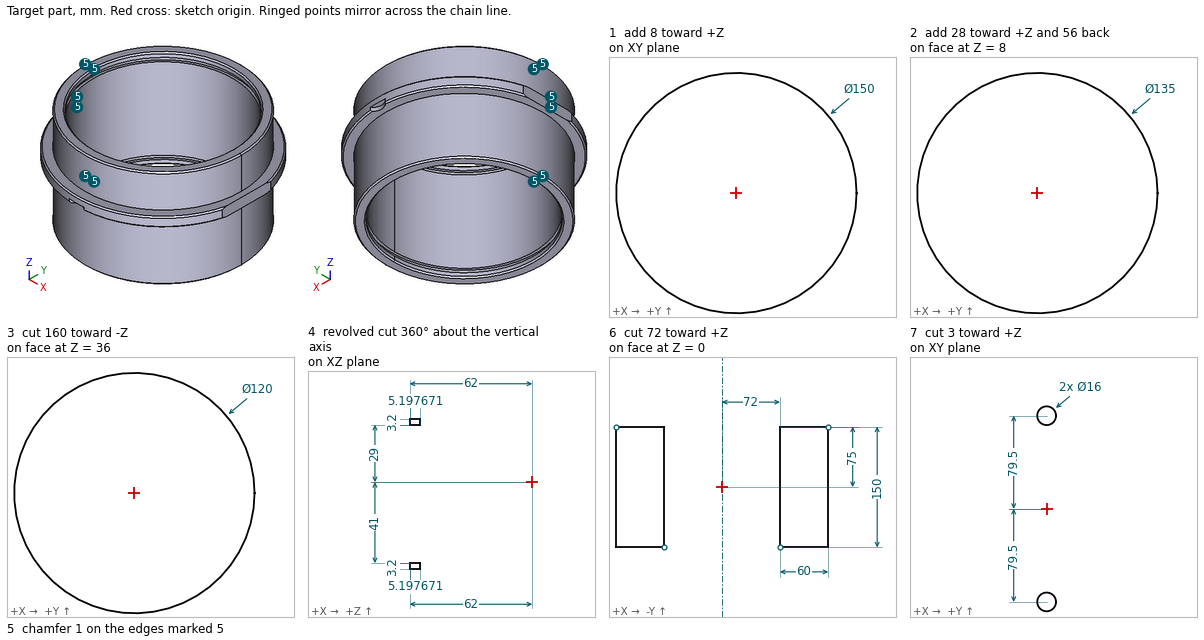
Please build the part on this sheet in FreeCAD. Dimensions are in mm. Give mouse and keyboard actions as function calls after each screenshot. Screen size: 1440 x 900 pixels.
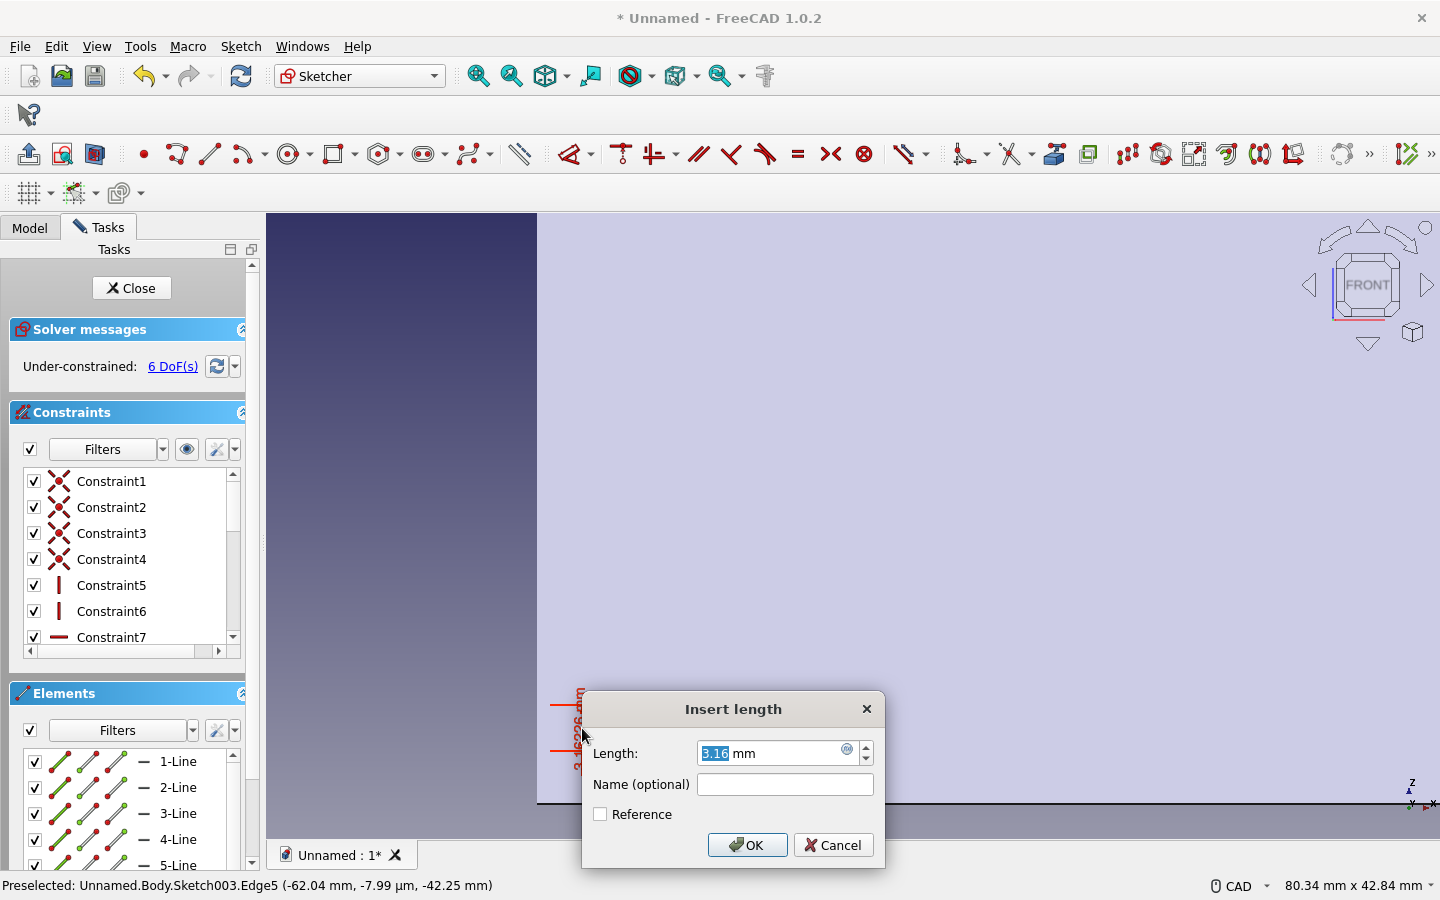
text(3.2)
key(Return)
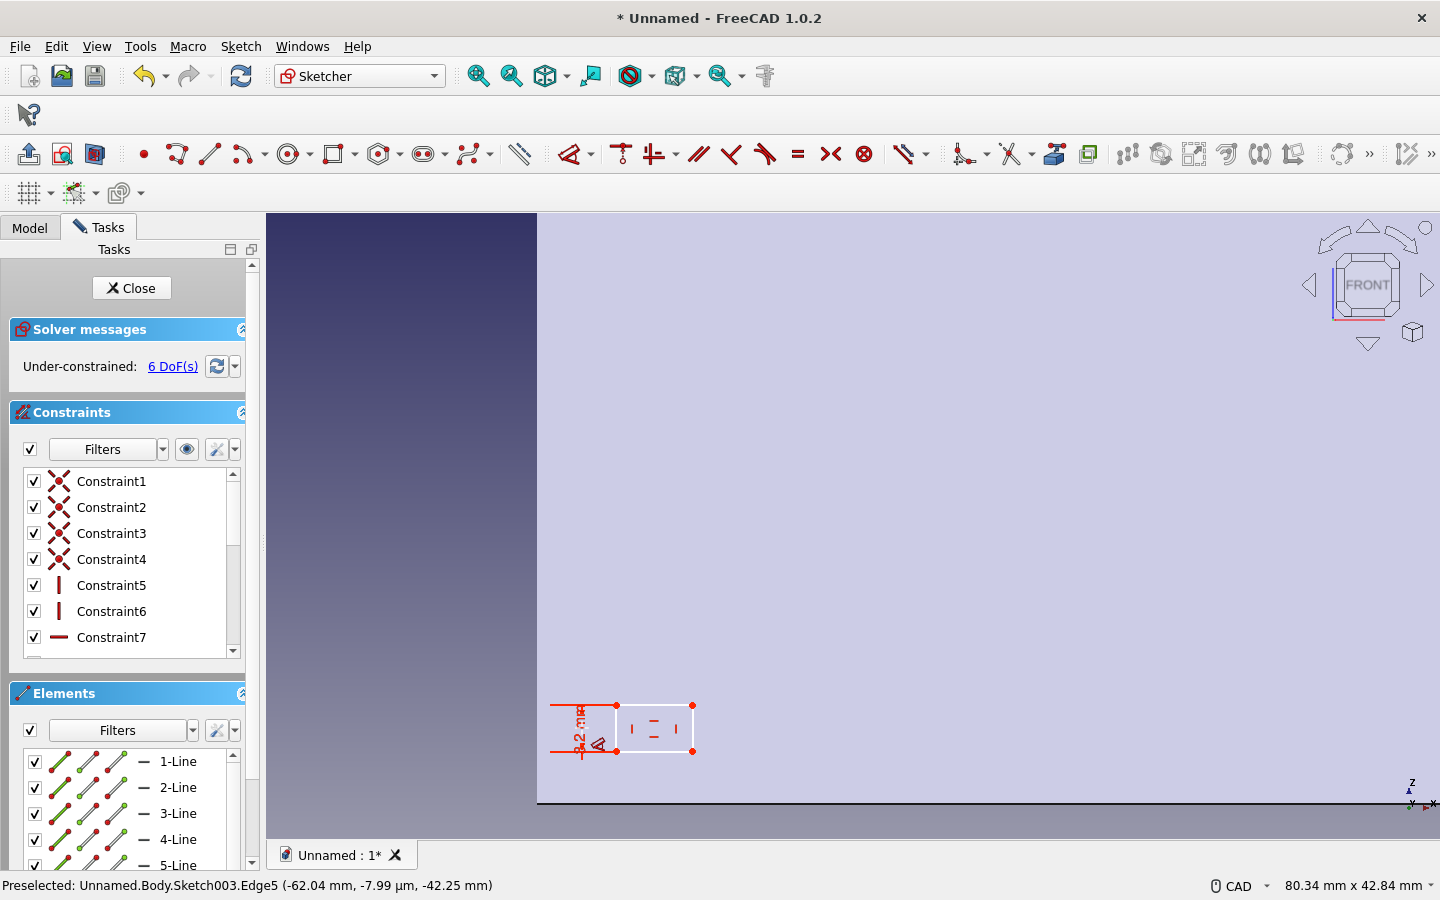
scroll(618, 721, down, 5)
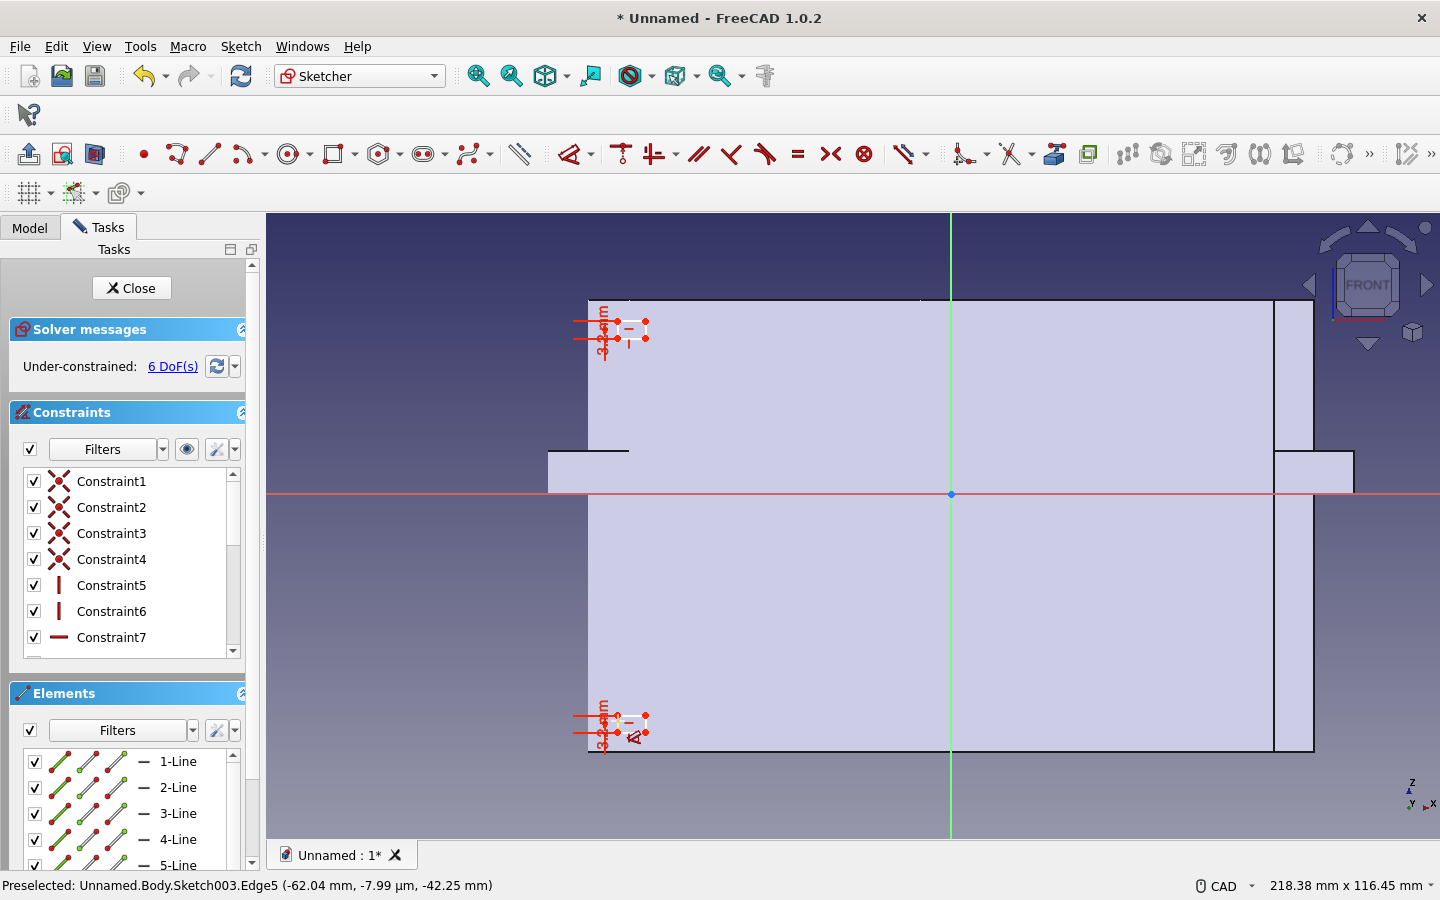
click(618, 321)
click(784, 287)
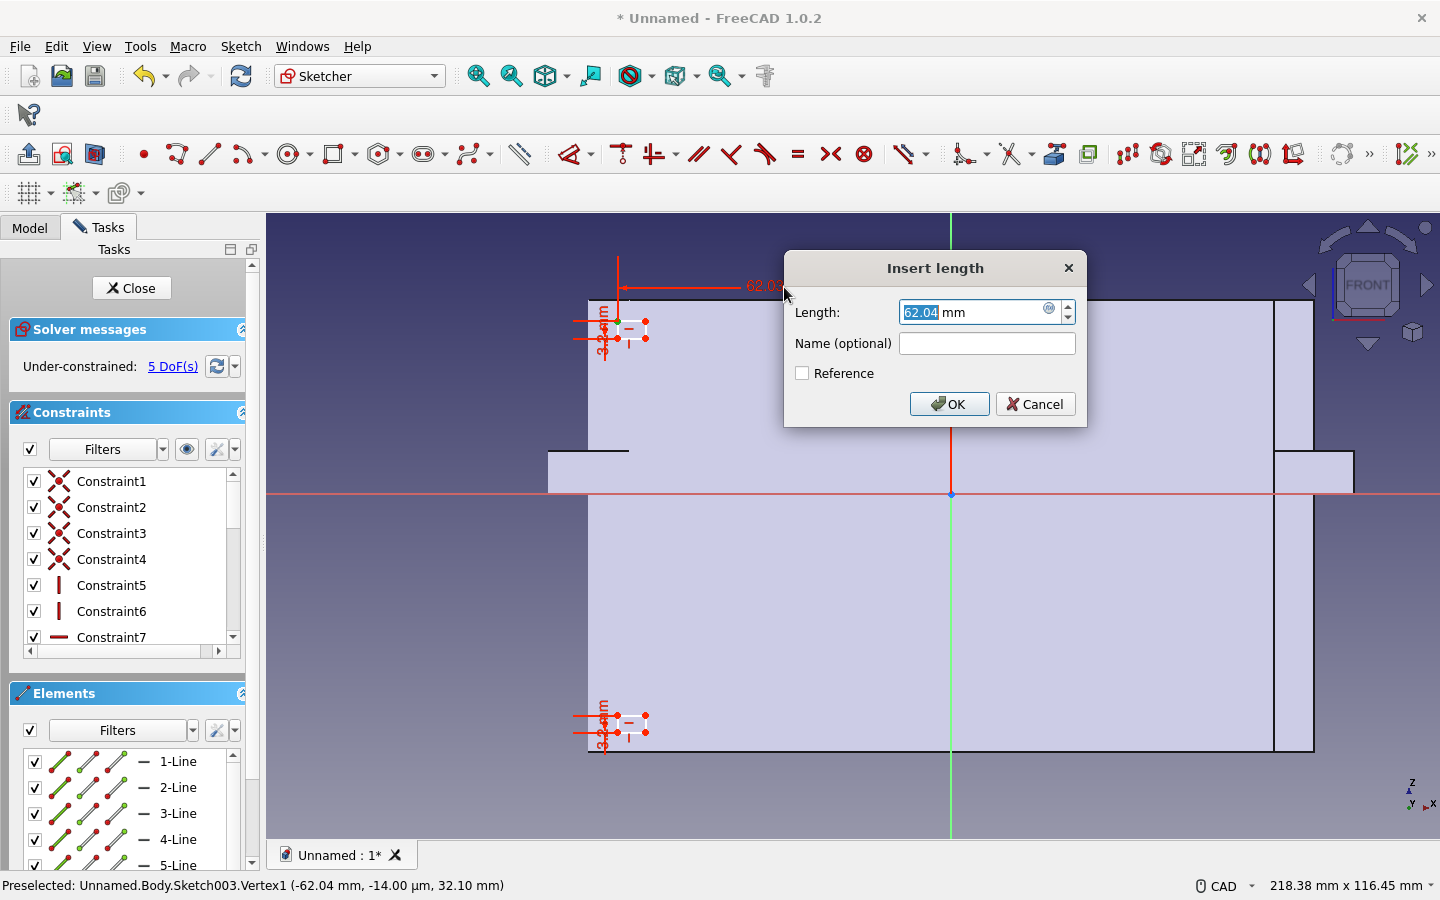
text(62)
key(Return)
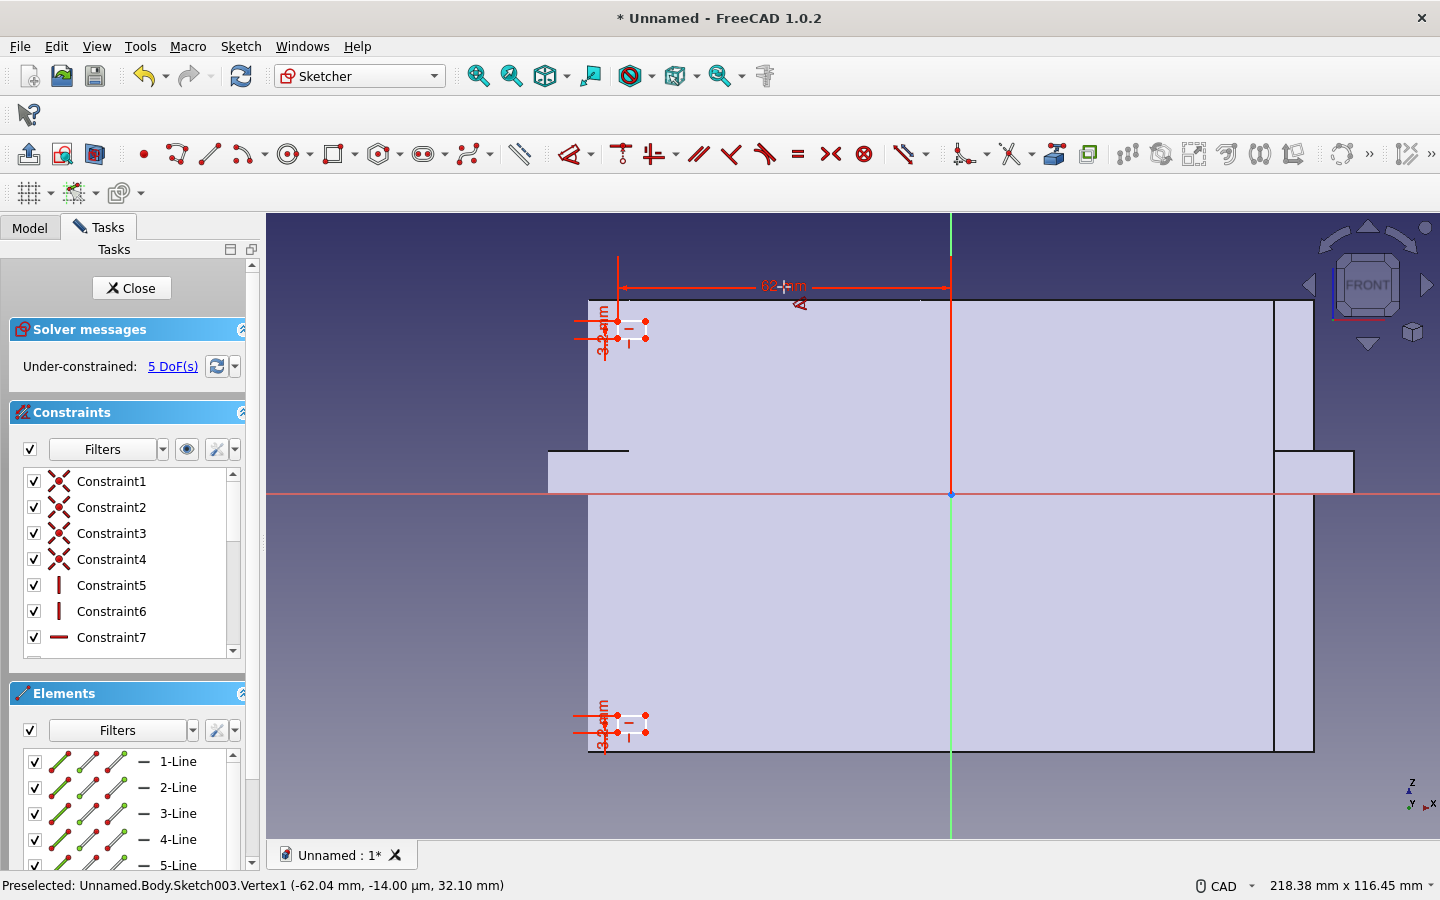
click(618, 339)
click(985, 416)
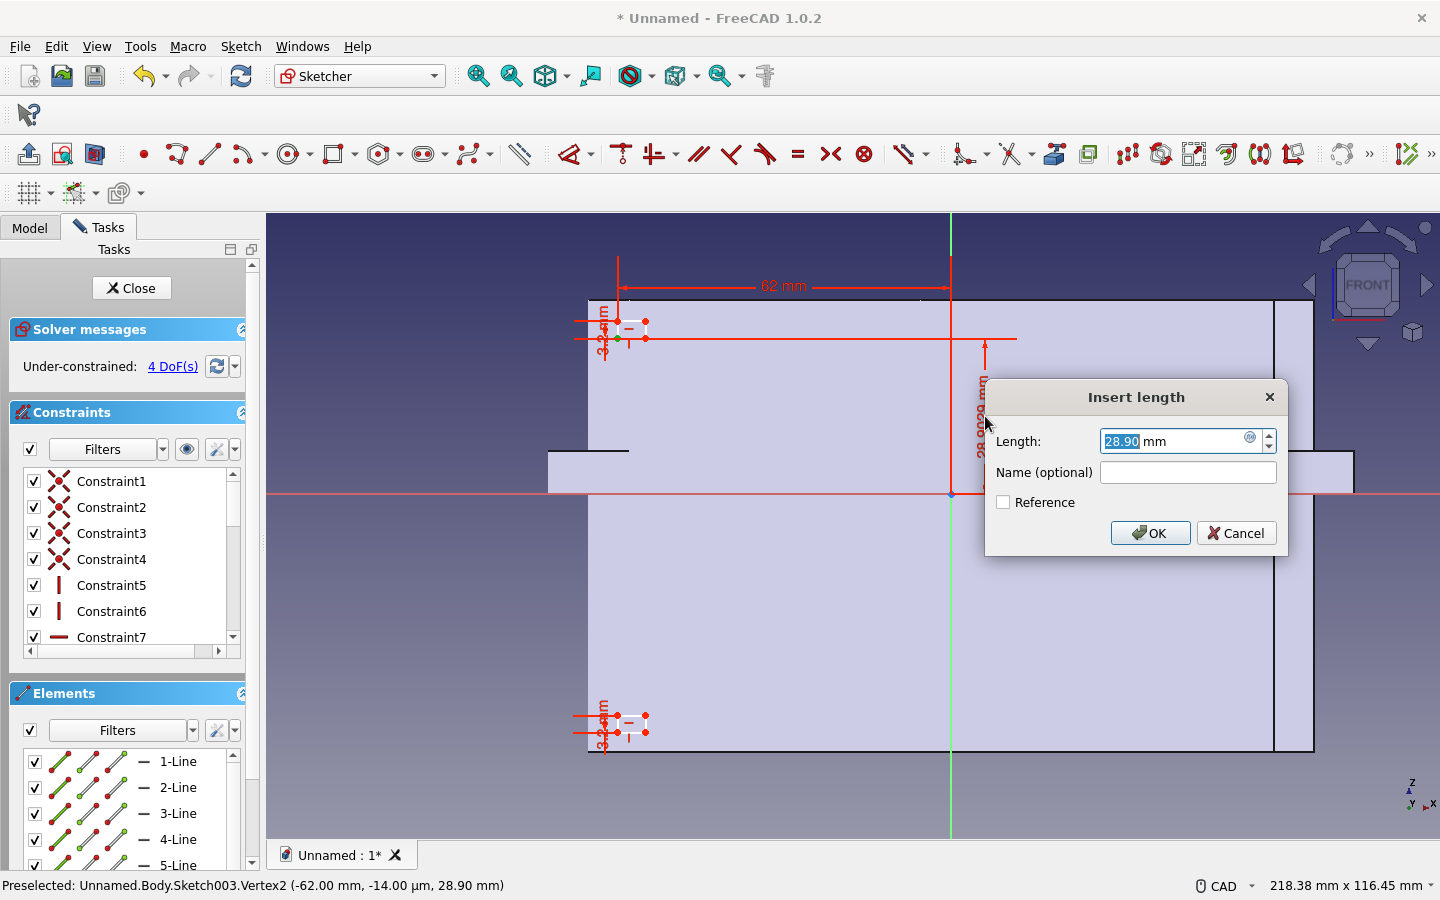
text(29)
key(Return)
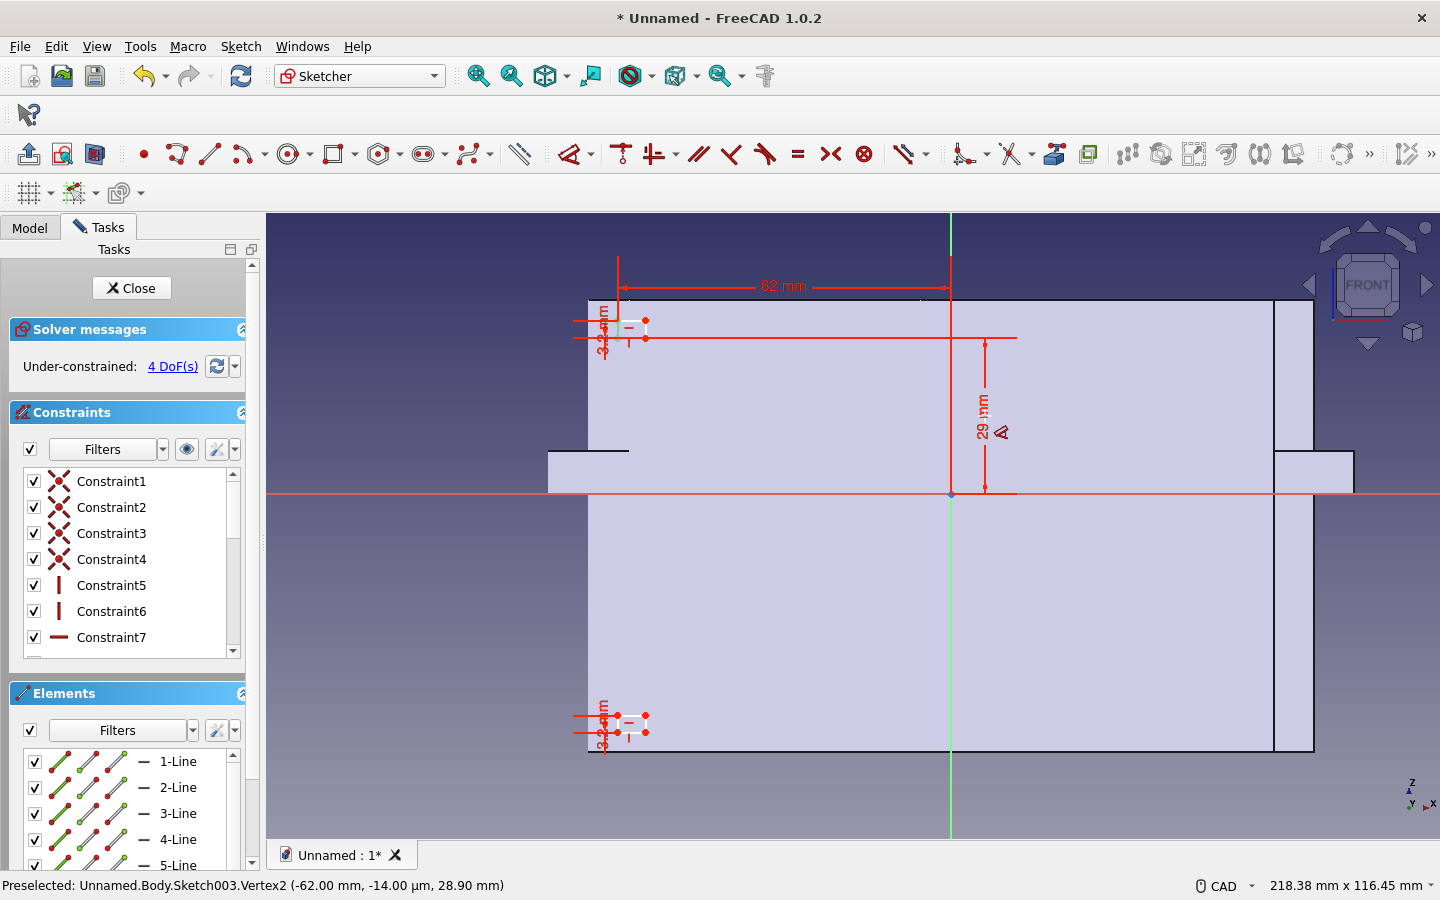
click(618, 716)
click(784, 750)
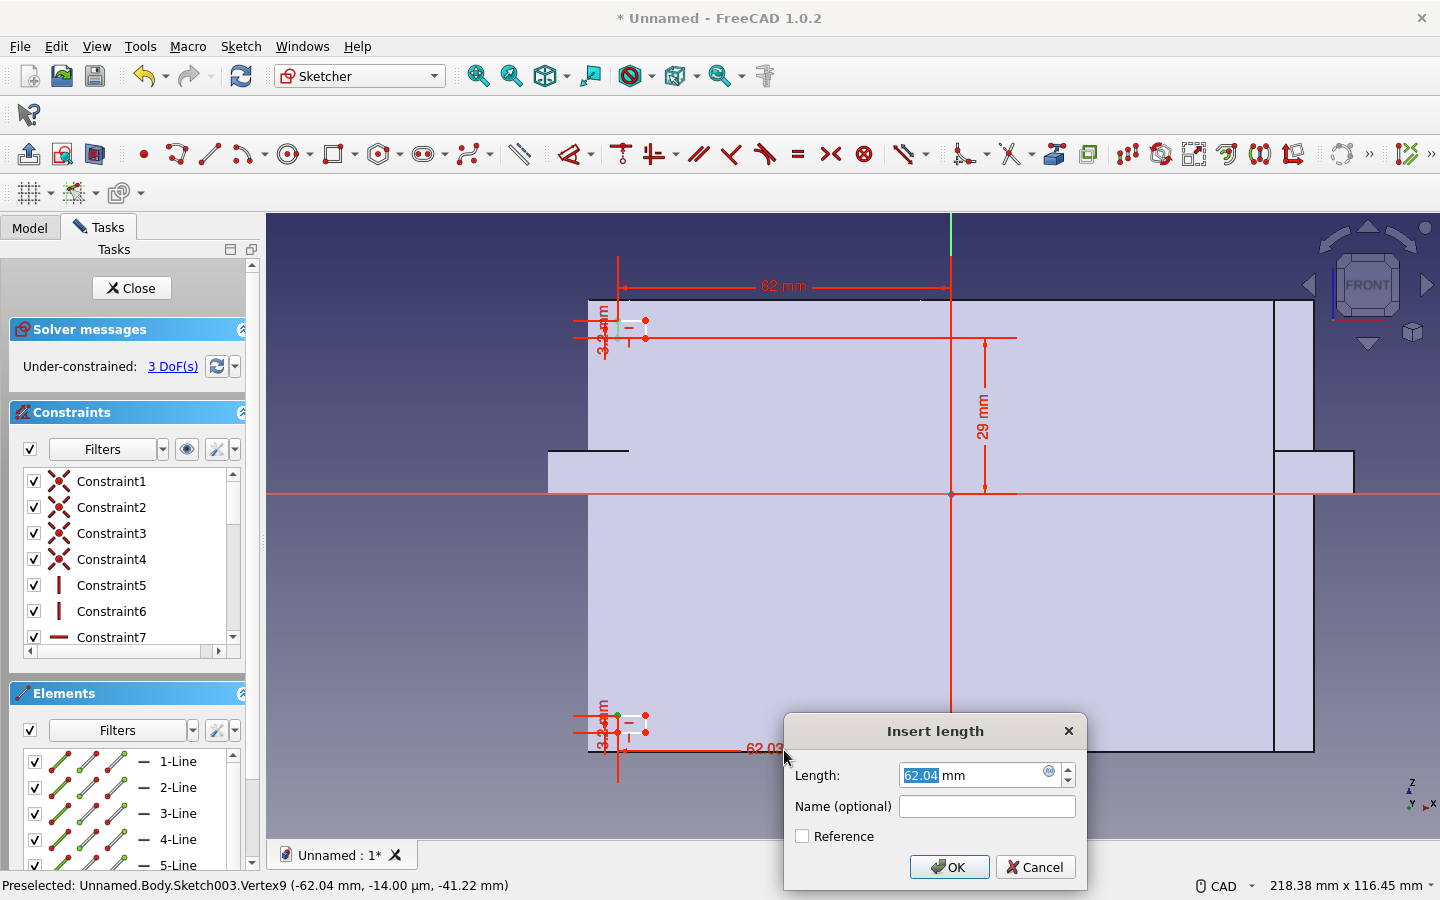
text(62)
key(Return)